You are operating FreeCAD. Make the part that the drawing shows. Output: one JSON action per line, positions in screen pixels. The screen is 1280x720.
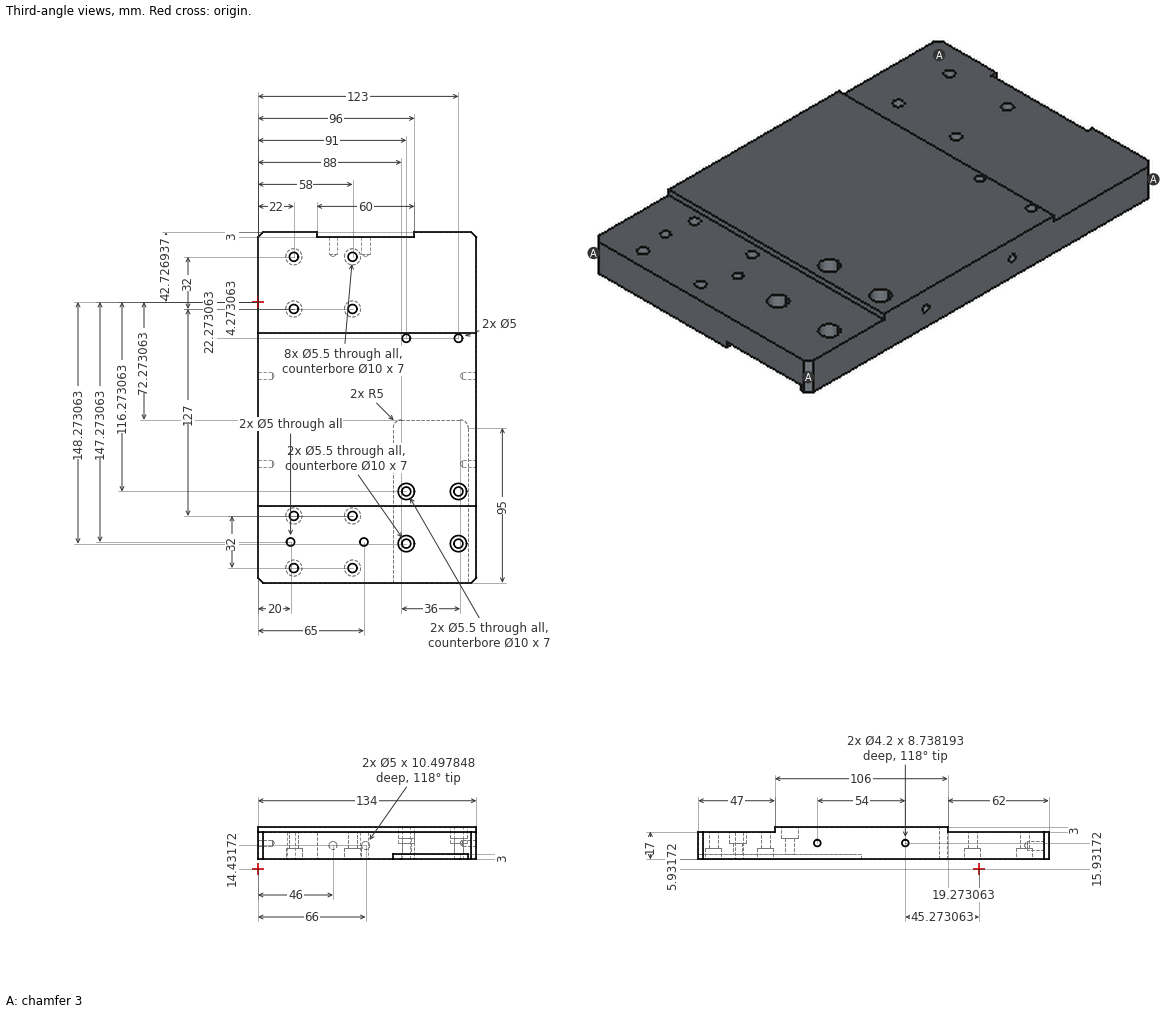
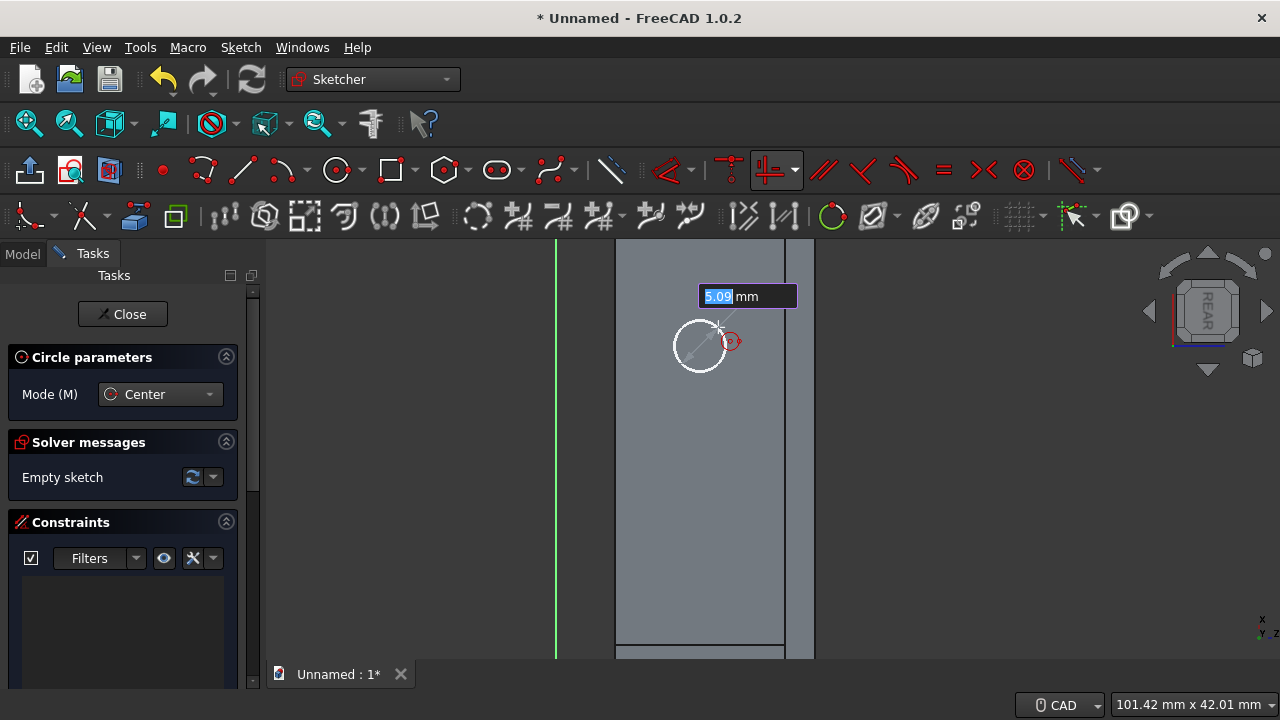
{"action": "type", "text": "5"}
{"action": "key", "text": "Return"}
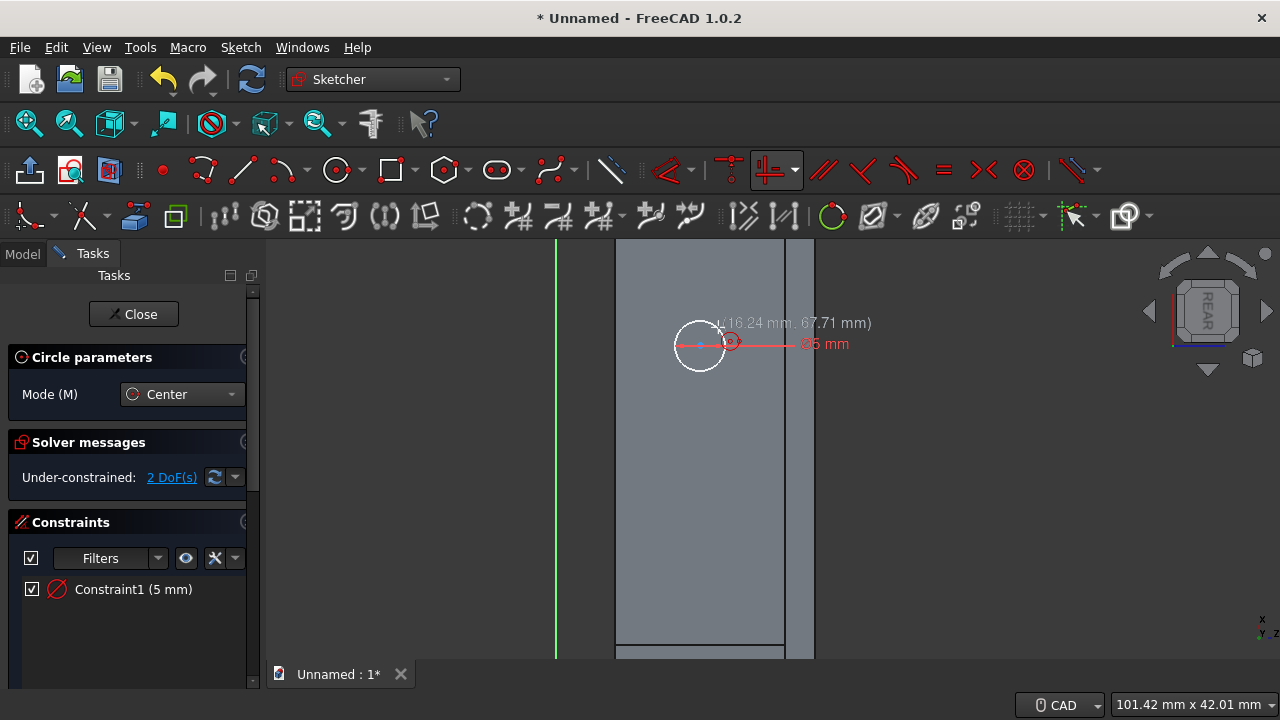
{"action": "left_click", "coordinate": [700, 545]}
{"action": "mouse_move", "coordinate": [718, 527]}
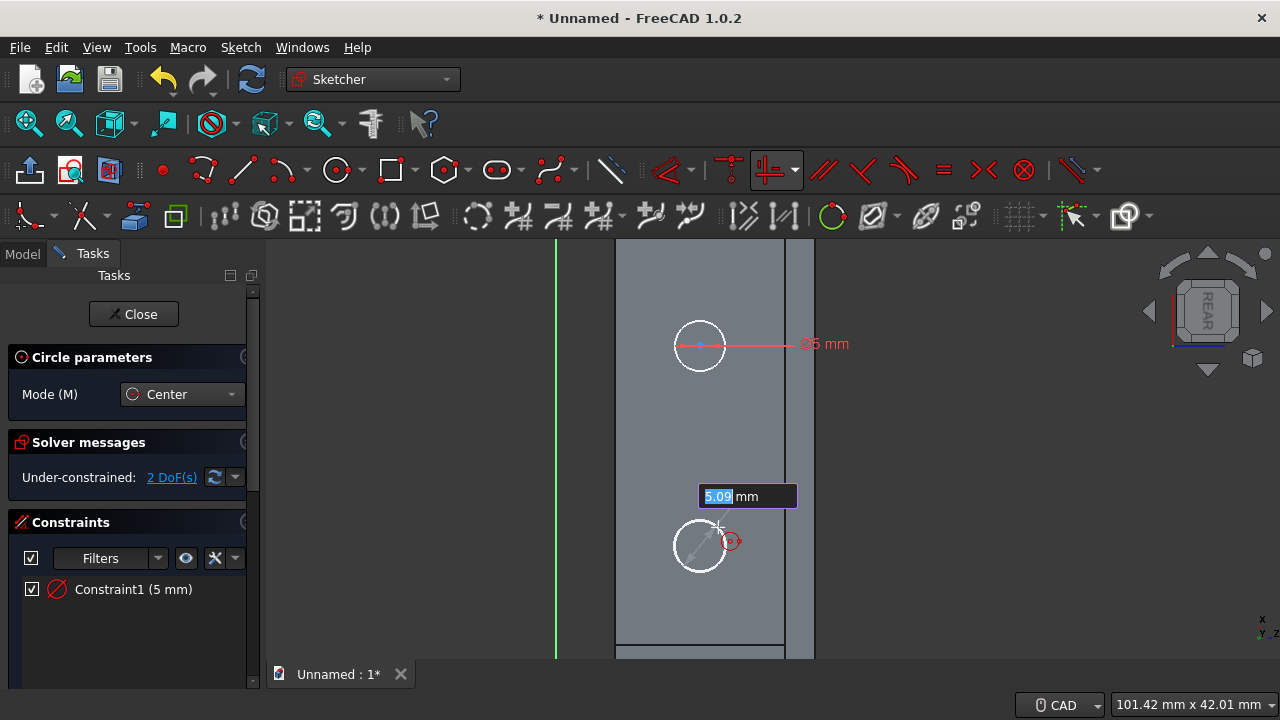
{"action": "type", "text": "5"}
{"action": "key", "text": "Return"}
{"action": "key", "text": "Escape"}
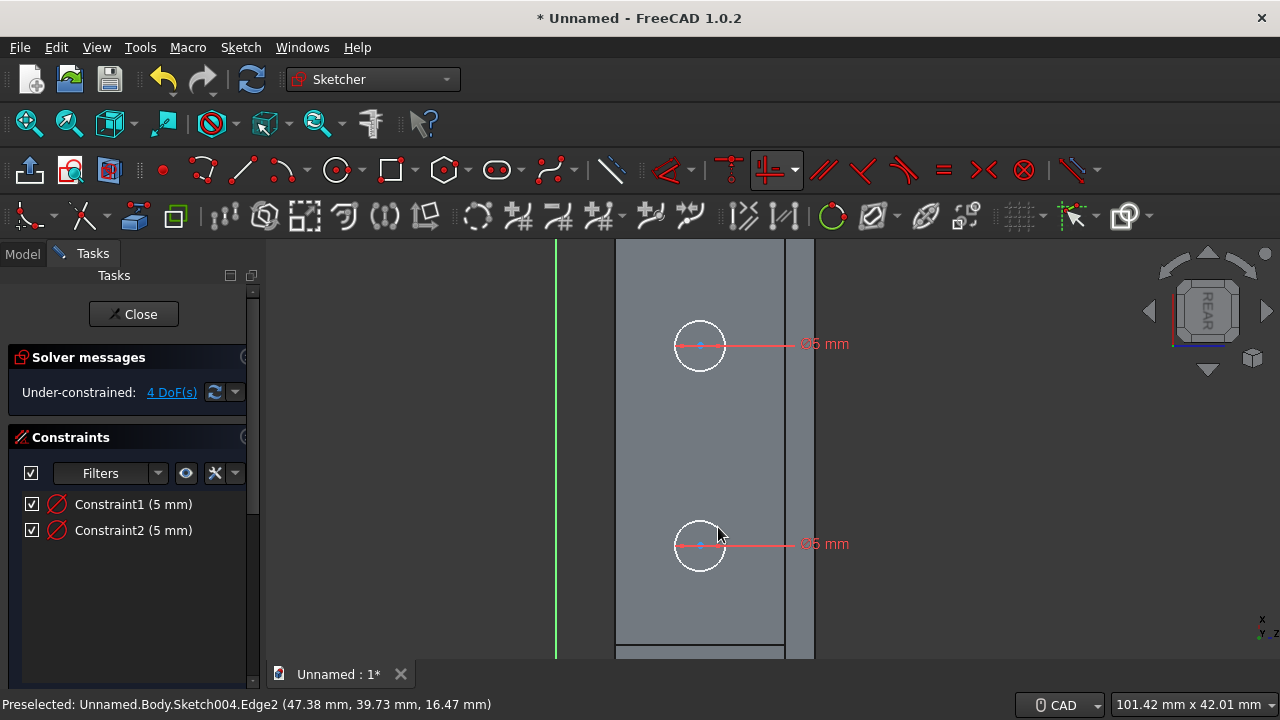
{"action": "left_click", "coordinate": [700, 346]}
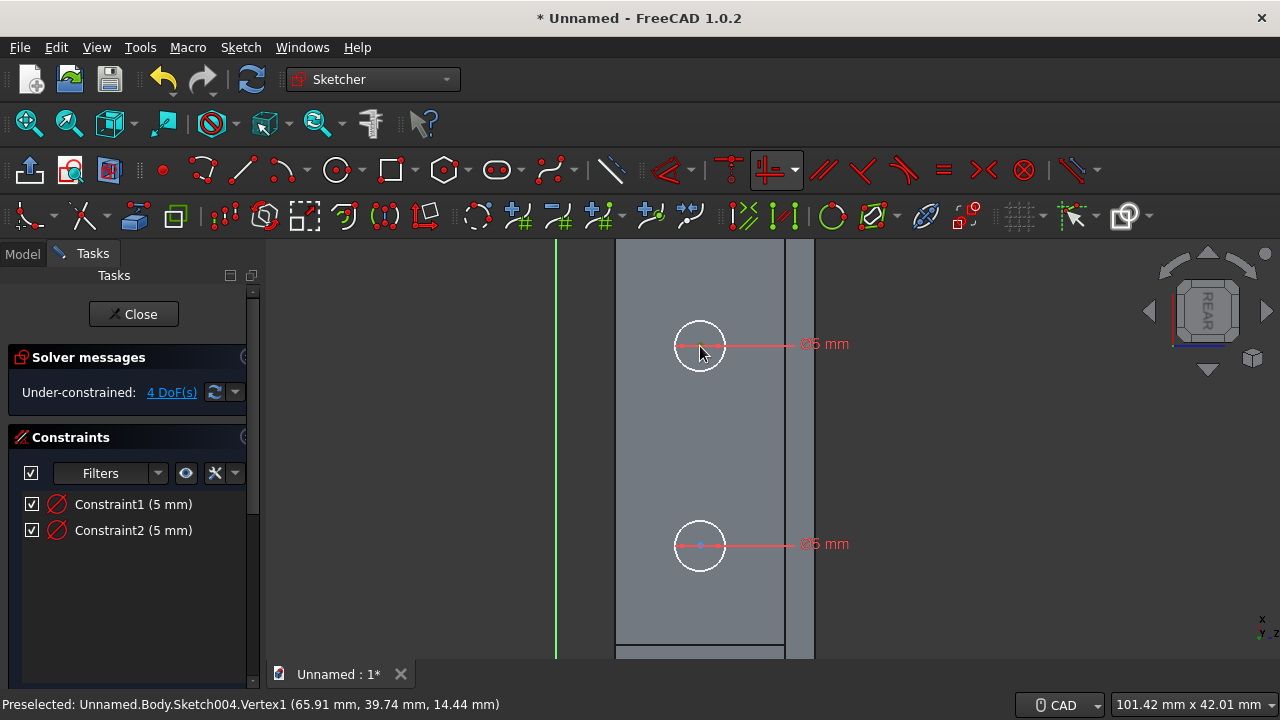
{"action": "left_click", "coordinate": [700, 546]}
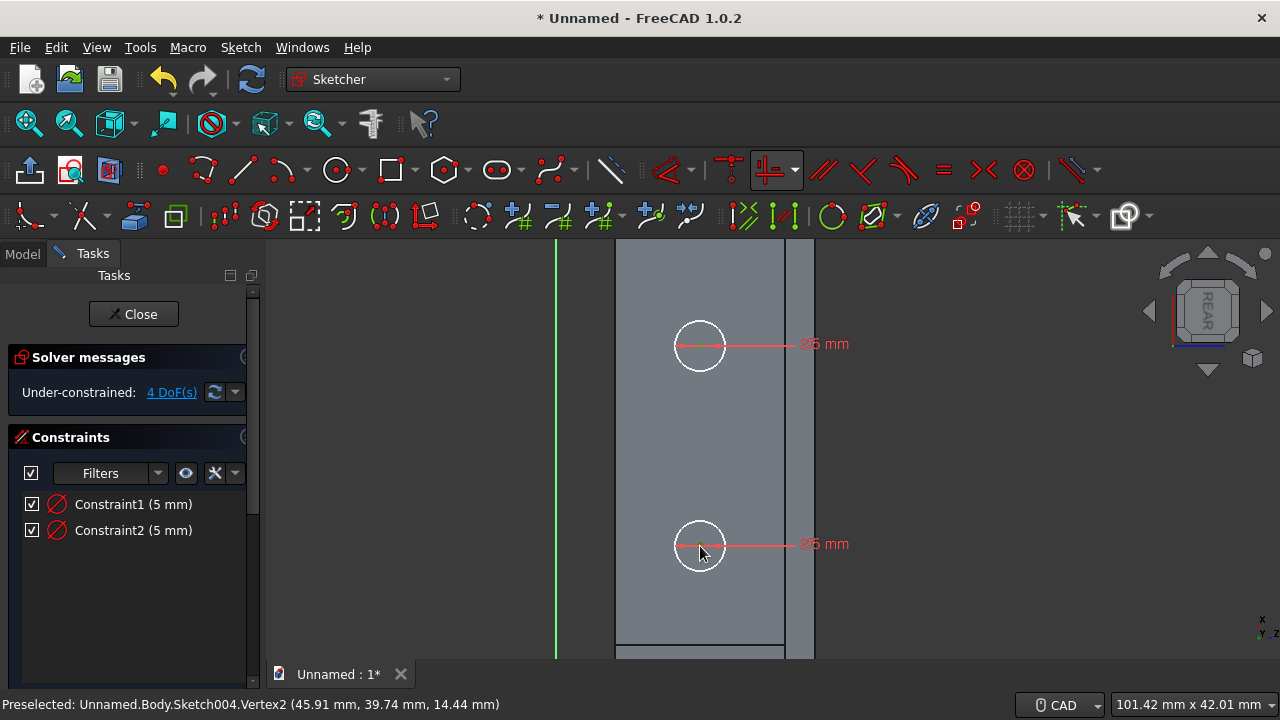
{"action": "left_click", "coordinate": [798, 170]}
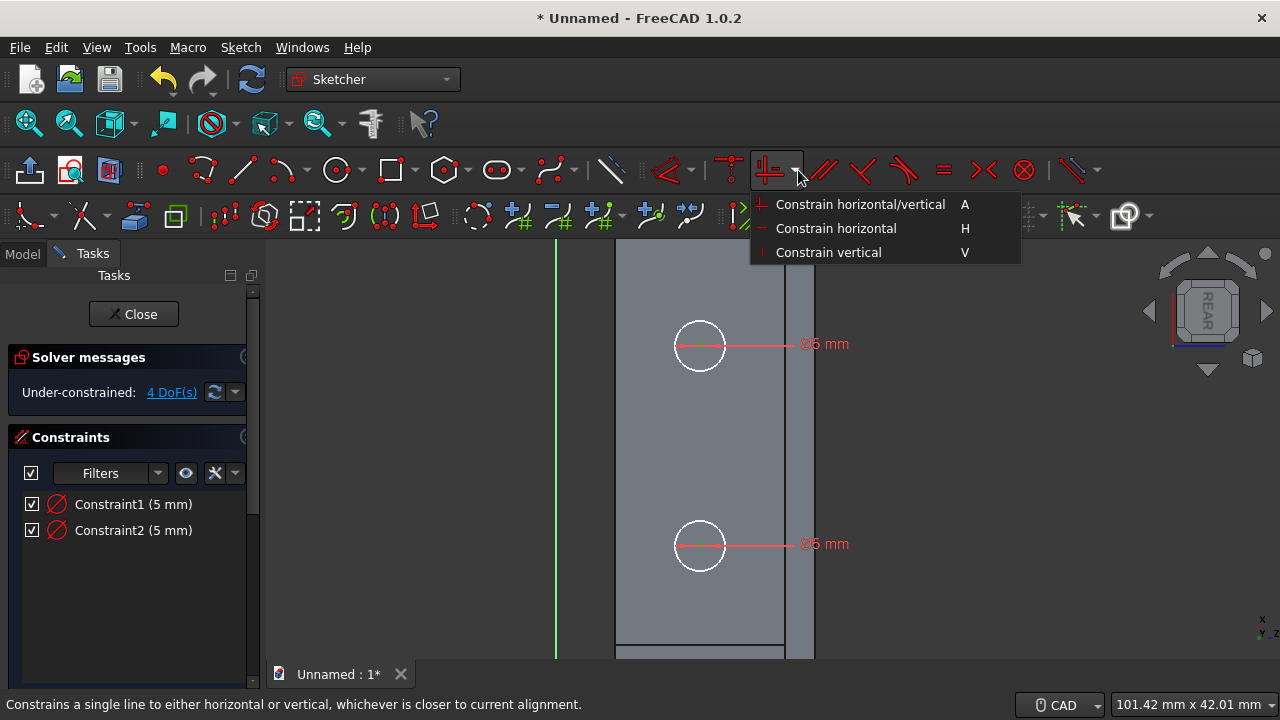
{"action": "left_click", "coordinate": [886, 252]}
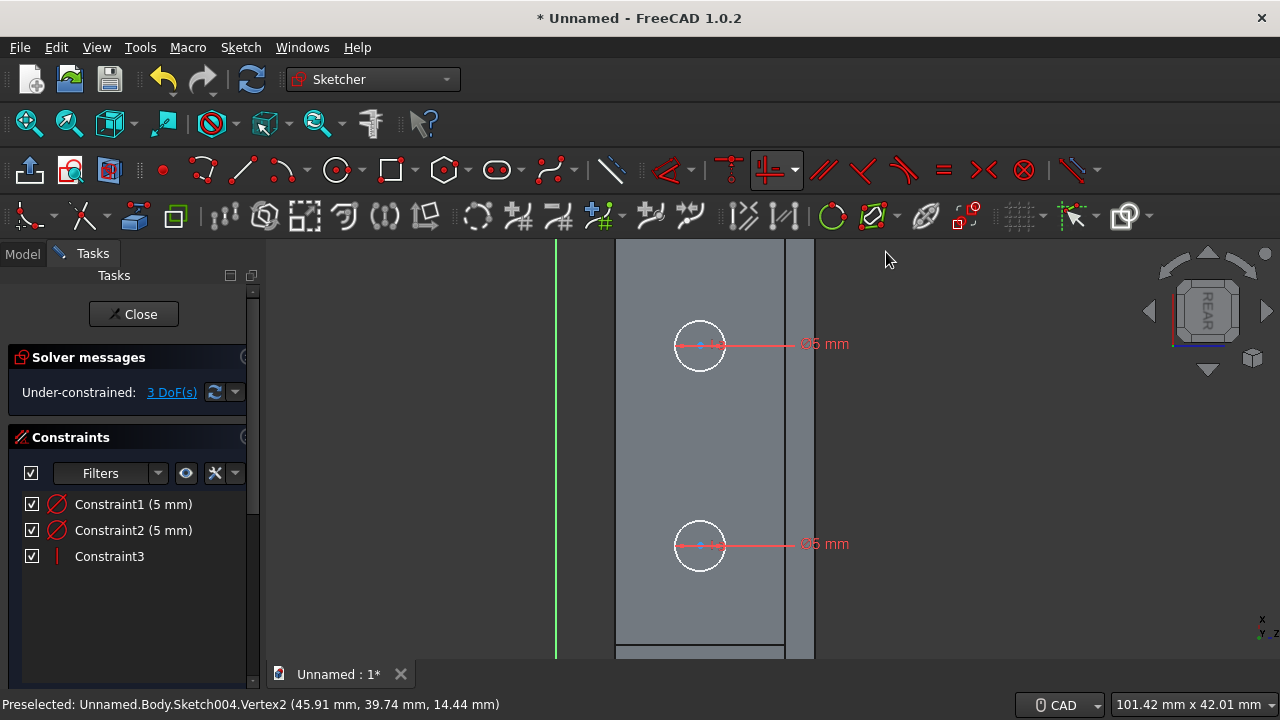
{"action": "left_click", "coordinate": [666, 170]}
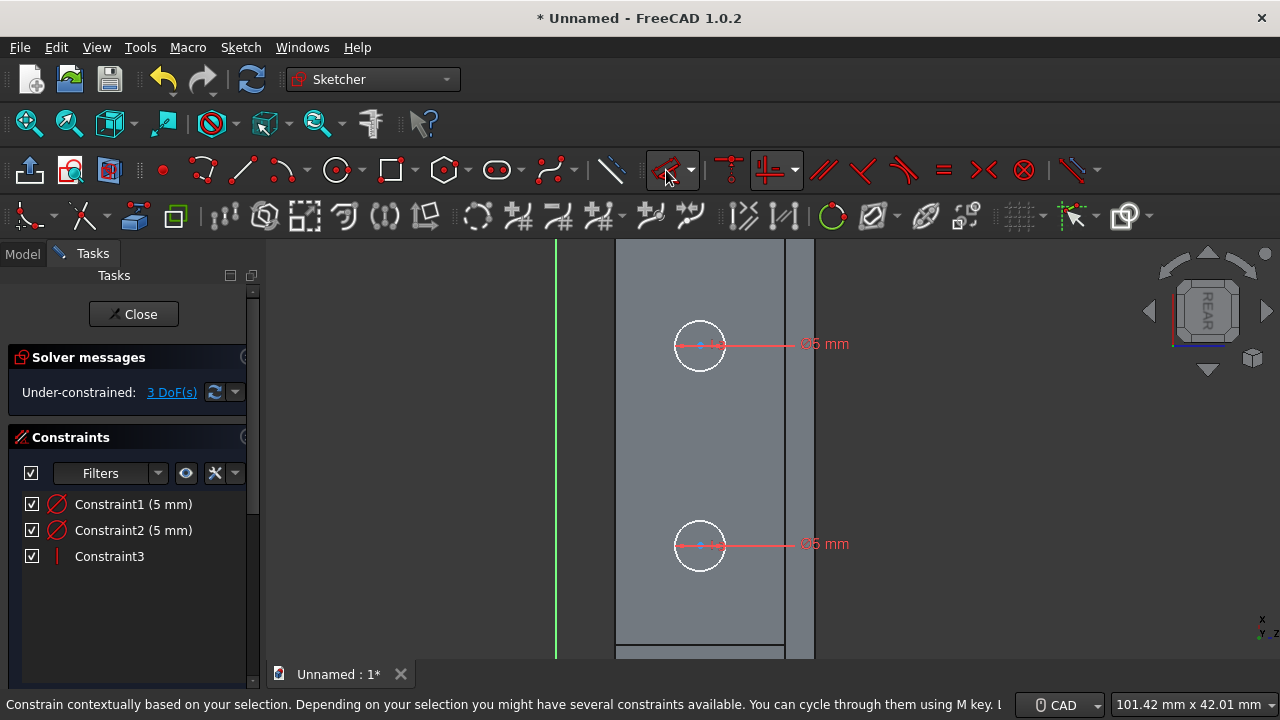
{"action": "left_click", "coordinate": [700, 346]}
{"action": "left_click", "coordinate": [522, 489]}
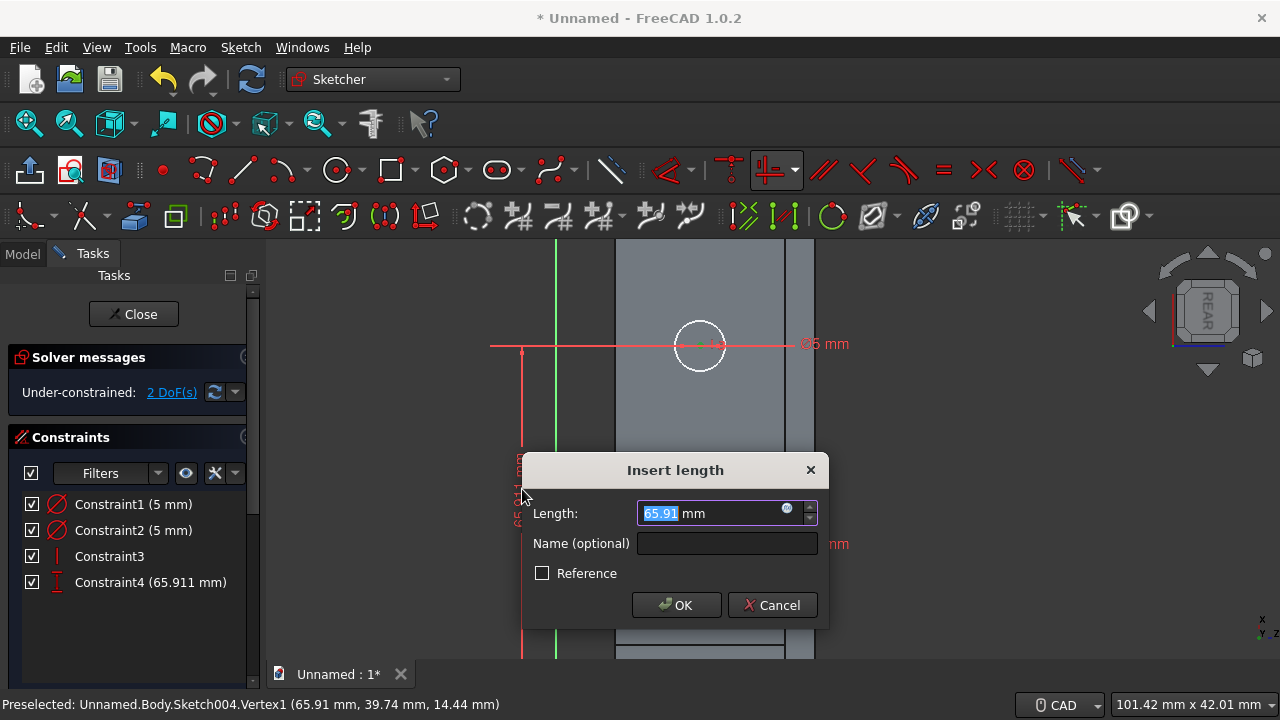
{"action": "type", "text": "66"}
{"action": "key", "text": "Return"}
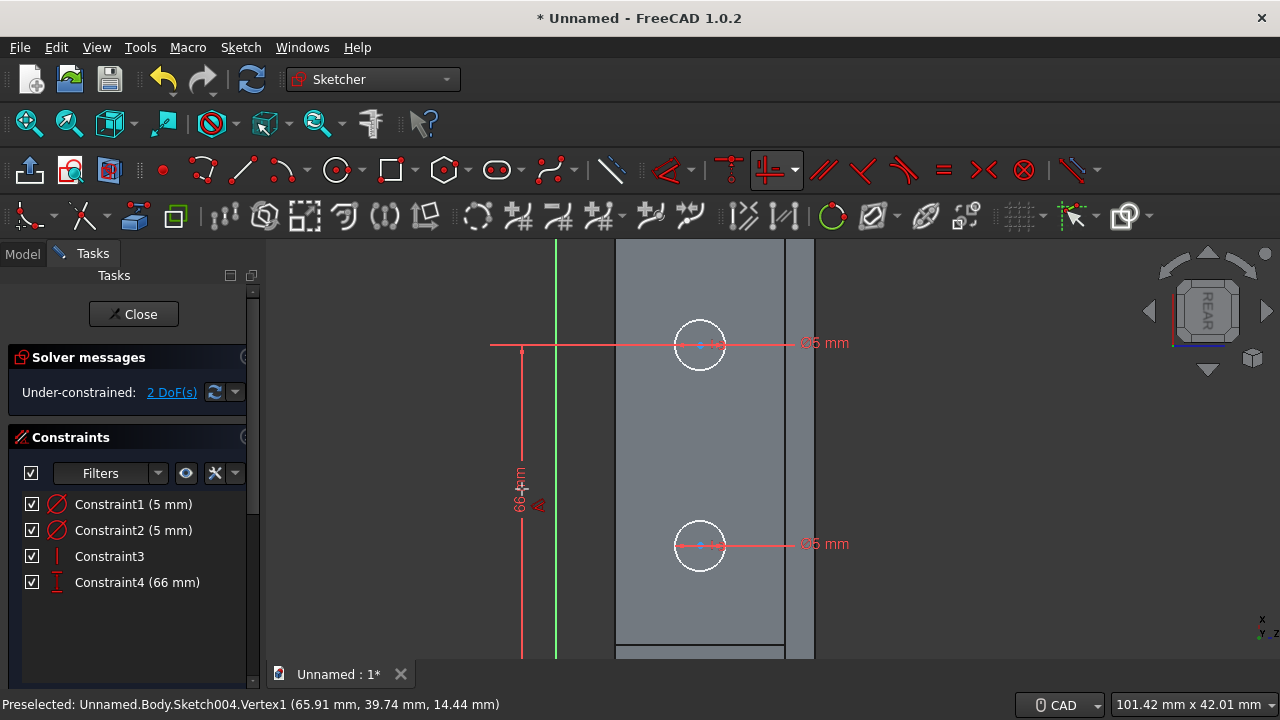
{"action": "left_click", "coordinate": [700, 546]}
{"action": "left_click", "coordinate": [522, 589]}